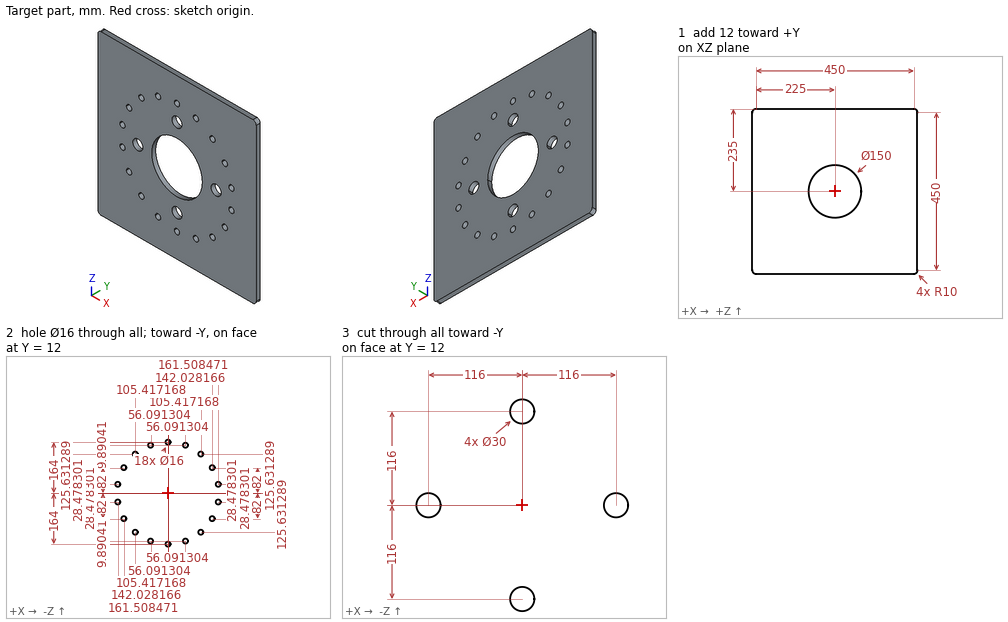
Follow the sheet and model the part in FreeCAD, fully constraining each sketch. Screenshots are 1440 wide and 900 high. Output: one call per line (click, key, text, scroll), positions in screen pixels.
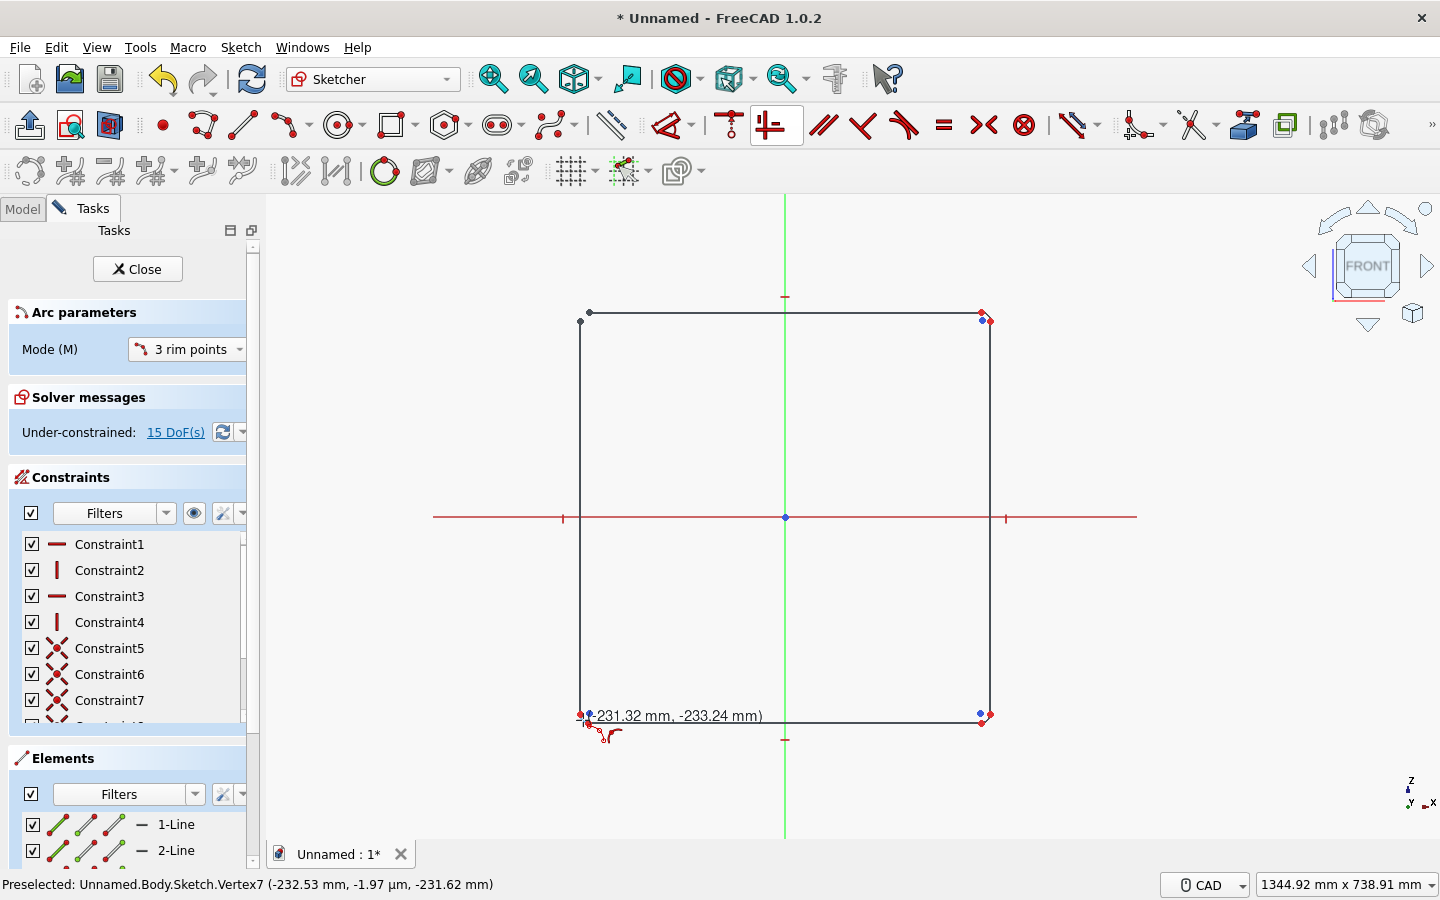
scroll(580, 321, up, 2)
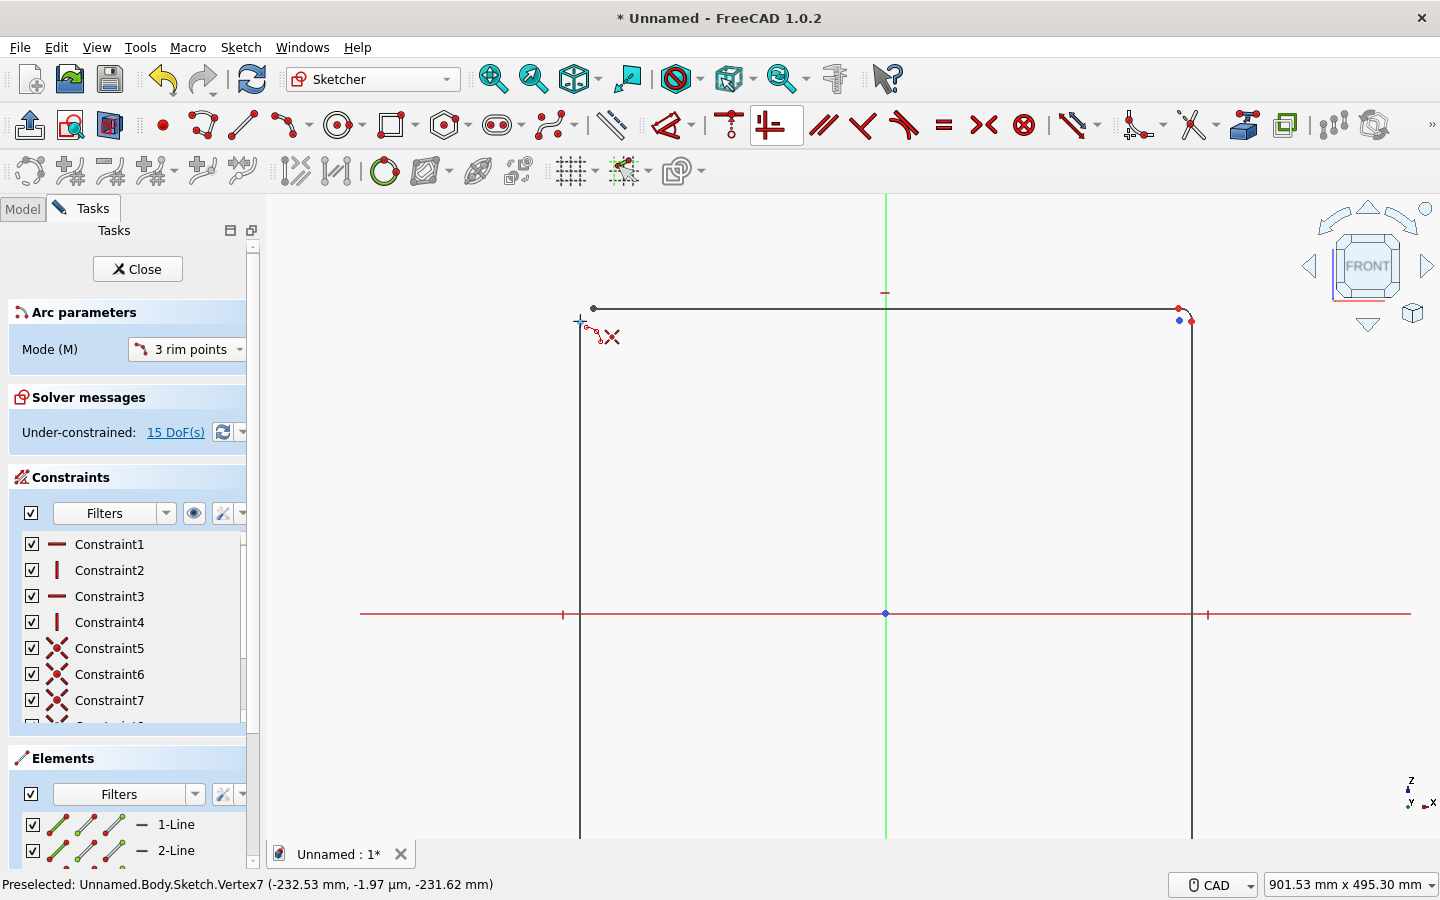
click(580, 322)
click(593, 309)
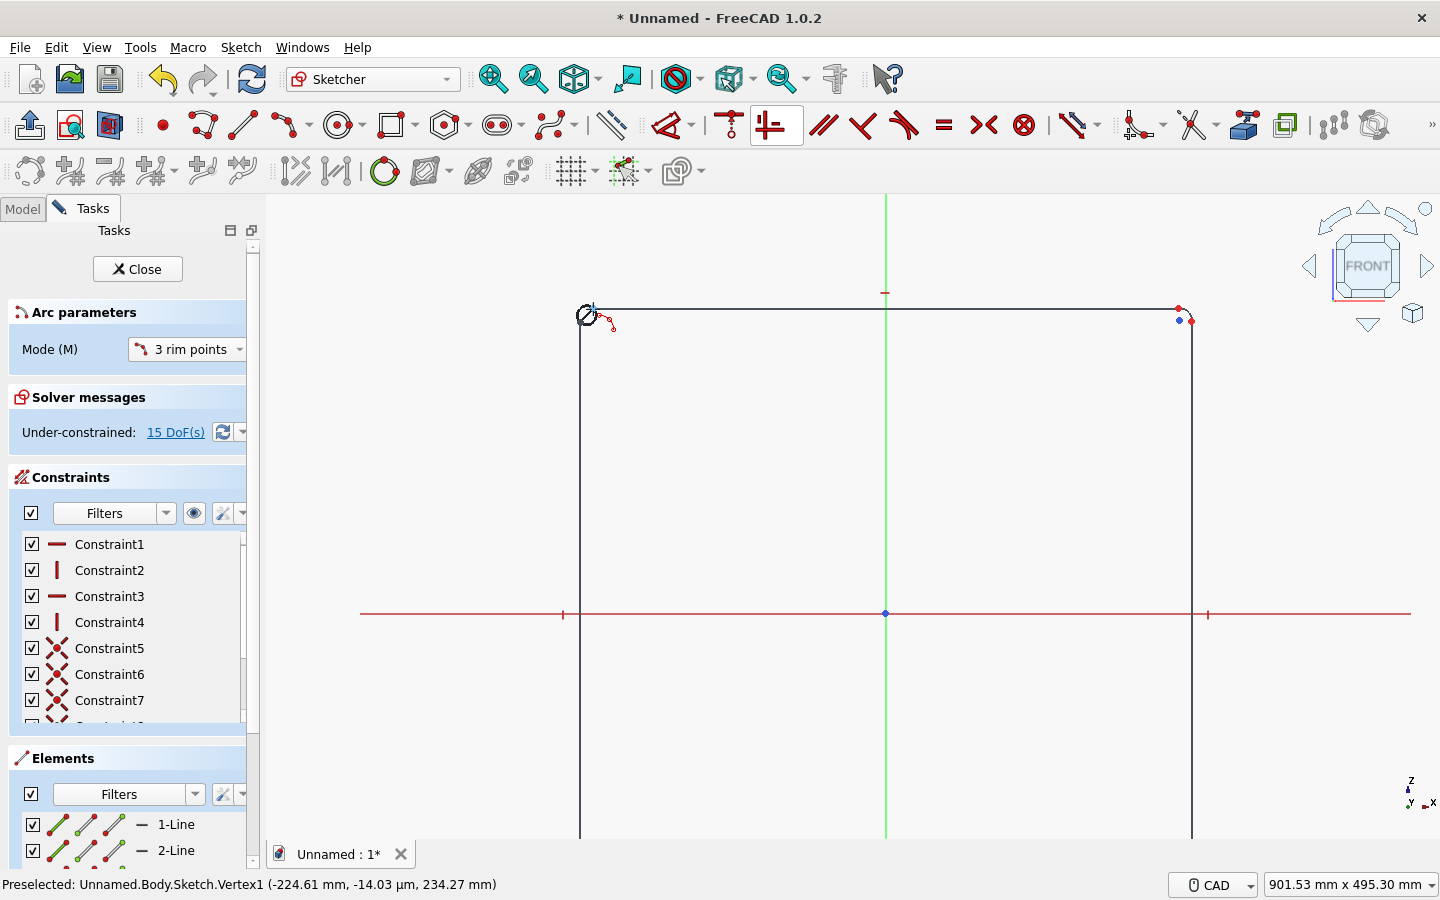
scroll(584, 311, up, 8)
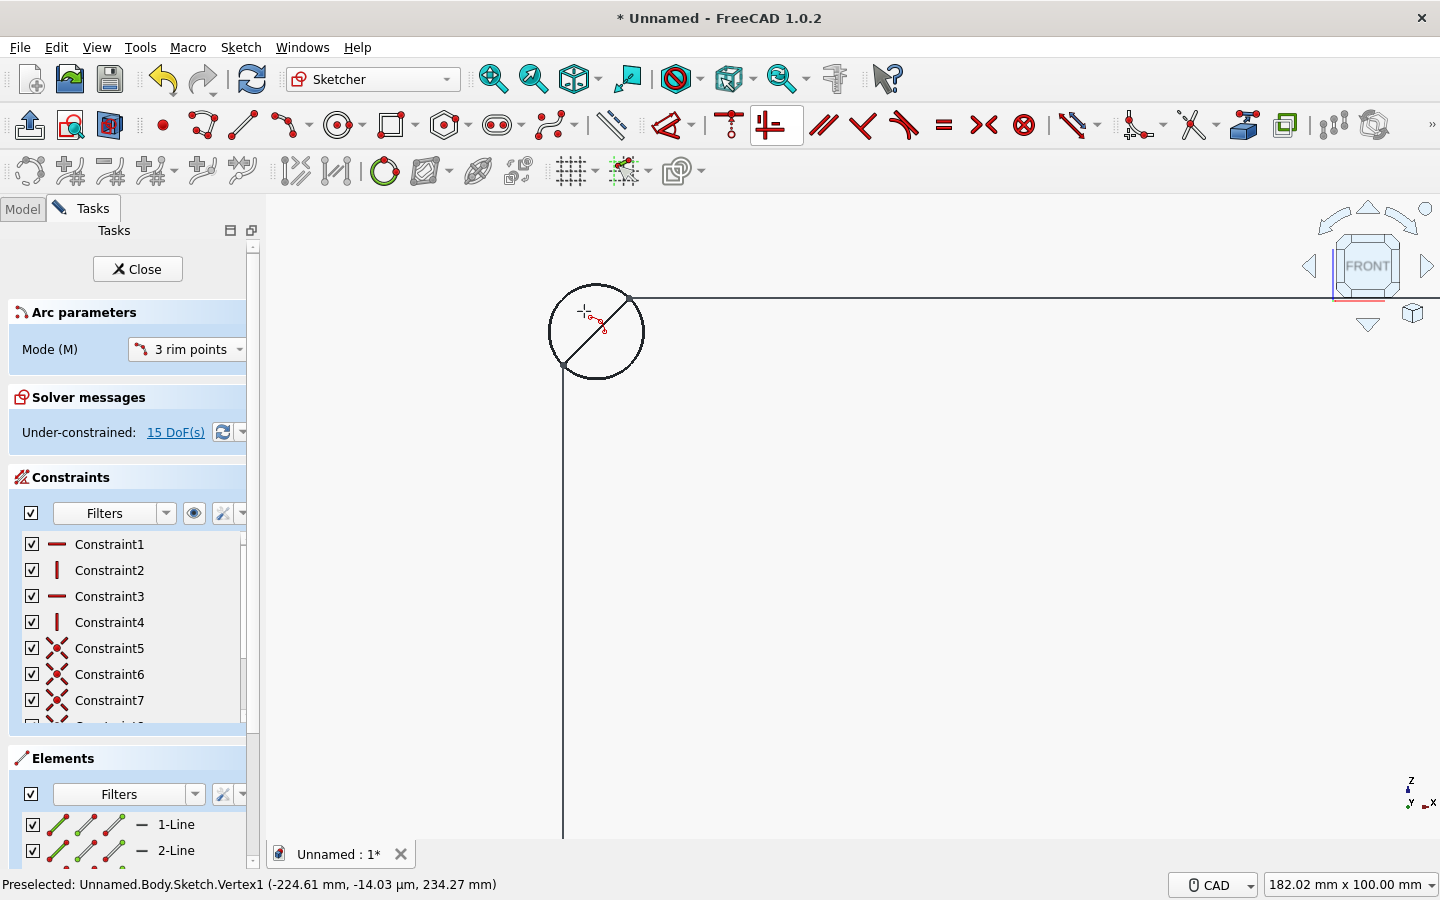
click(581, 313)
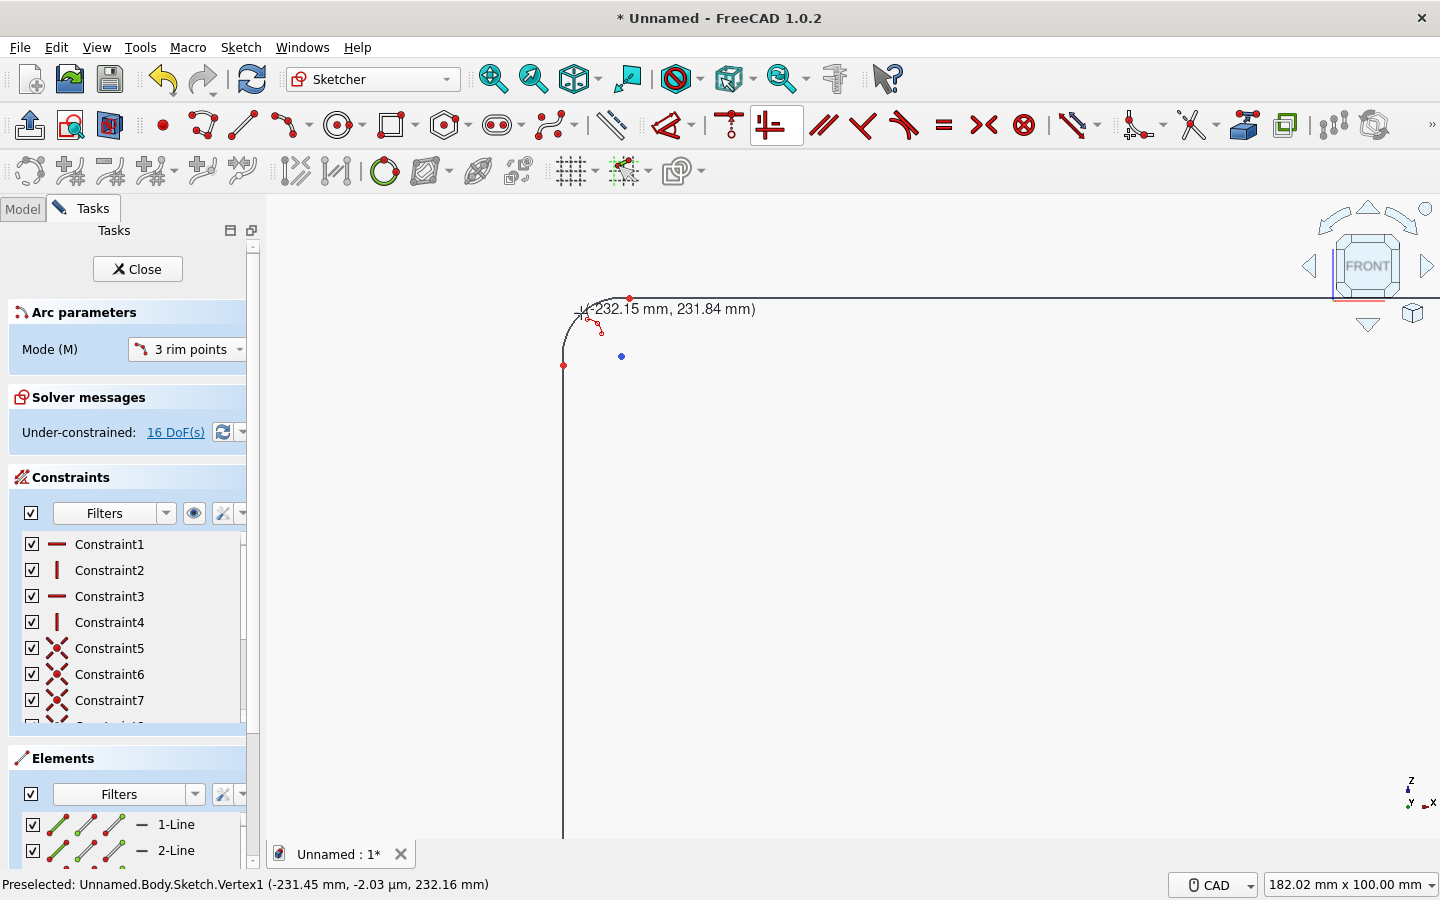
key(g)
key(c)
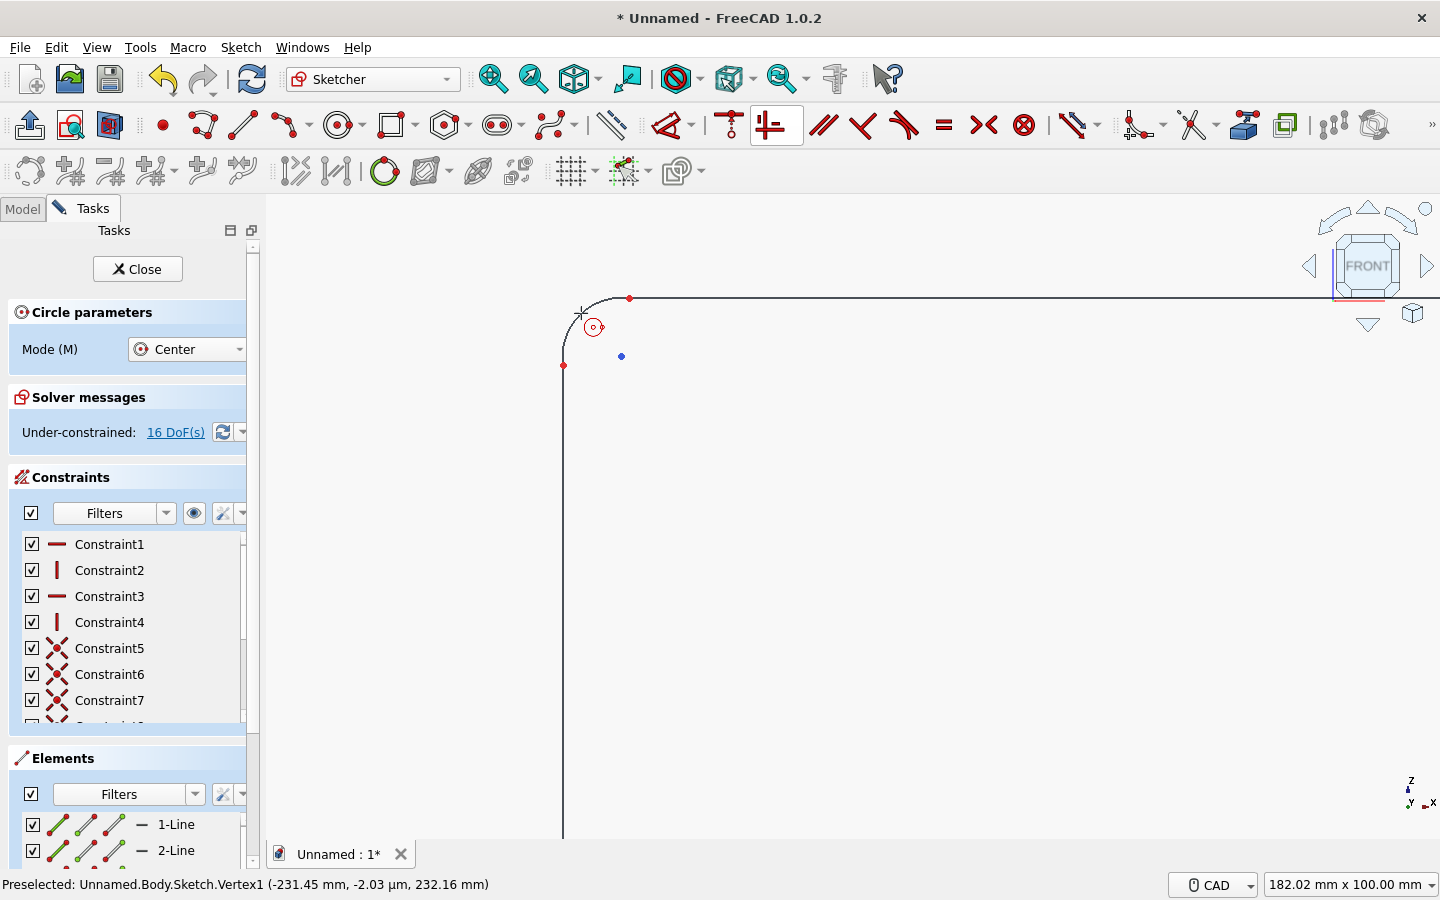
scroll(582, 314, down, 10)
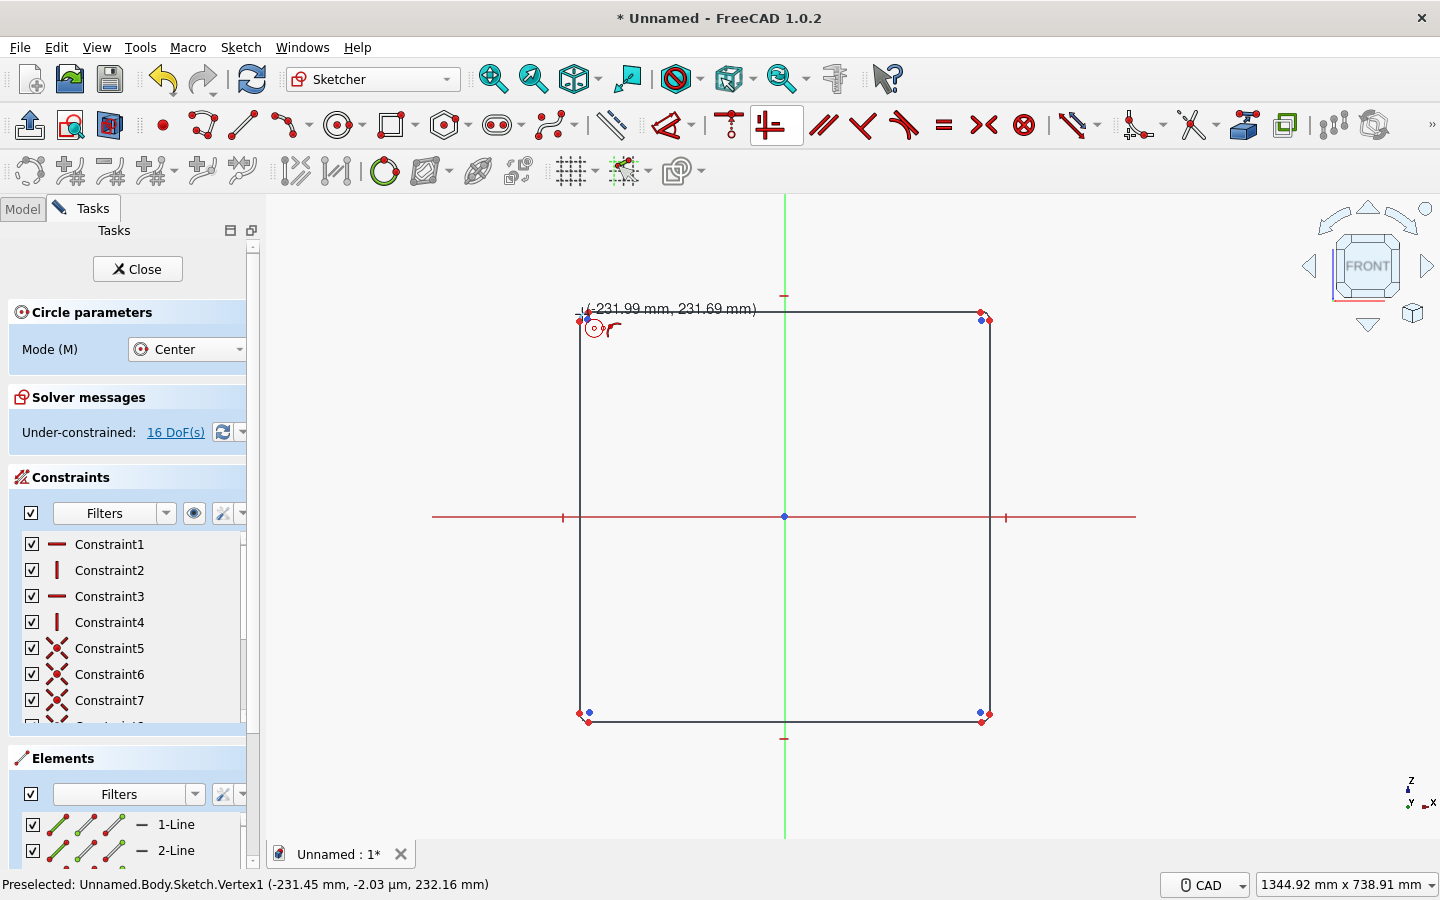
click(785, 517)
move(831, 470)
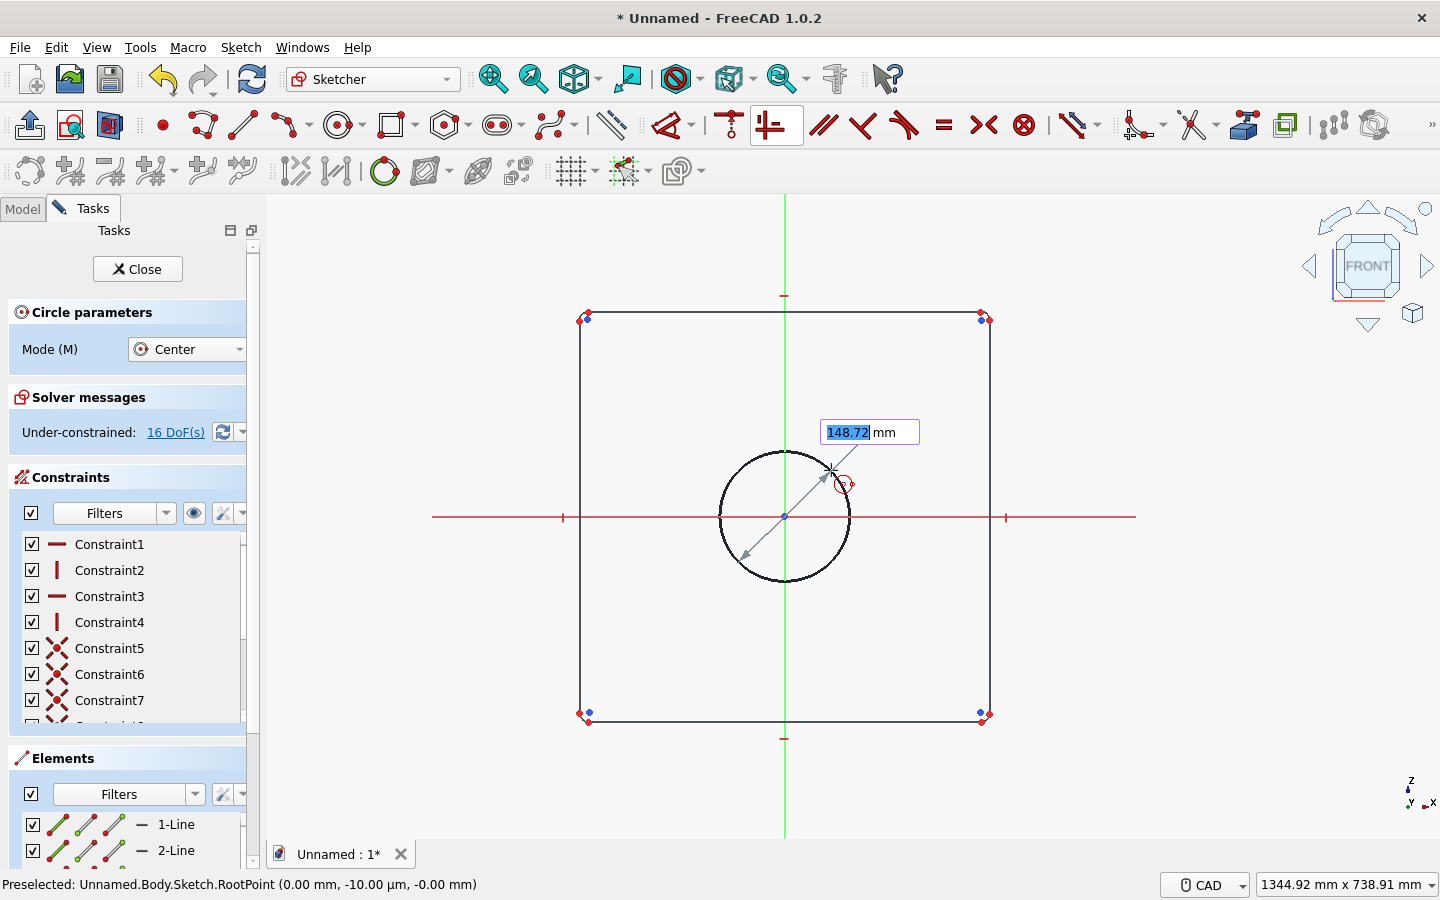
text(150)
key(Return)
key(Escape)